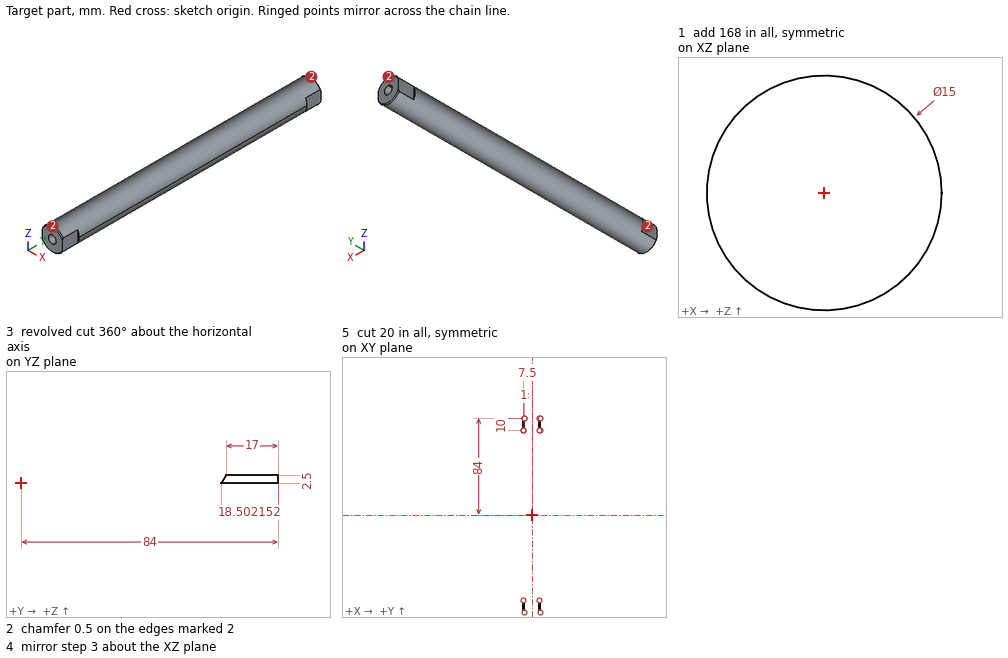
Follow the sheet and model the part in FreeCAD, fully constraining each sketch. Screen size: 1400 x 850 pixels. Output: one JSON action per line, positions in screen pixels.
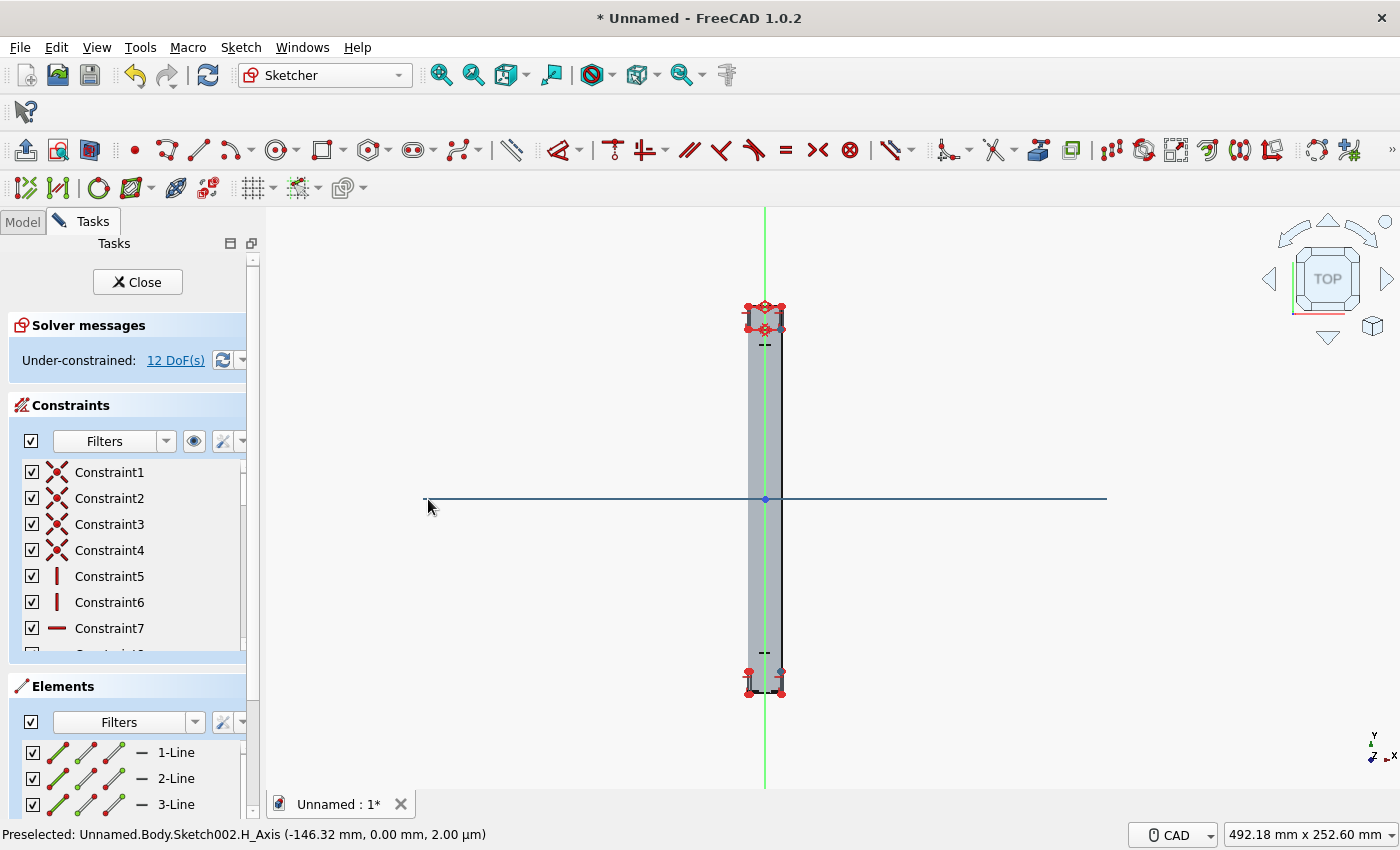
{"action": "left_click", "coordinate": [818, 150]}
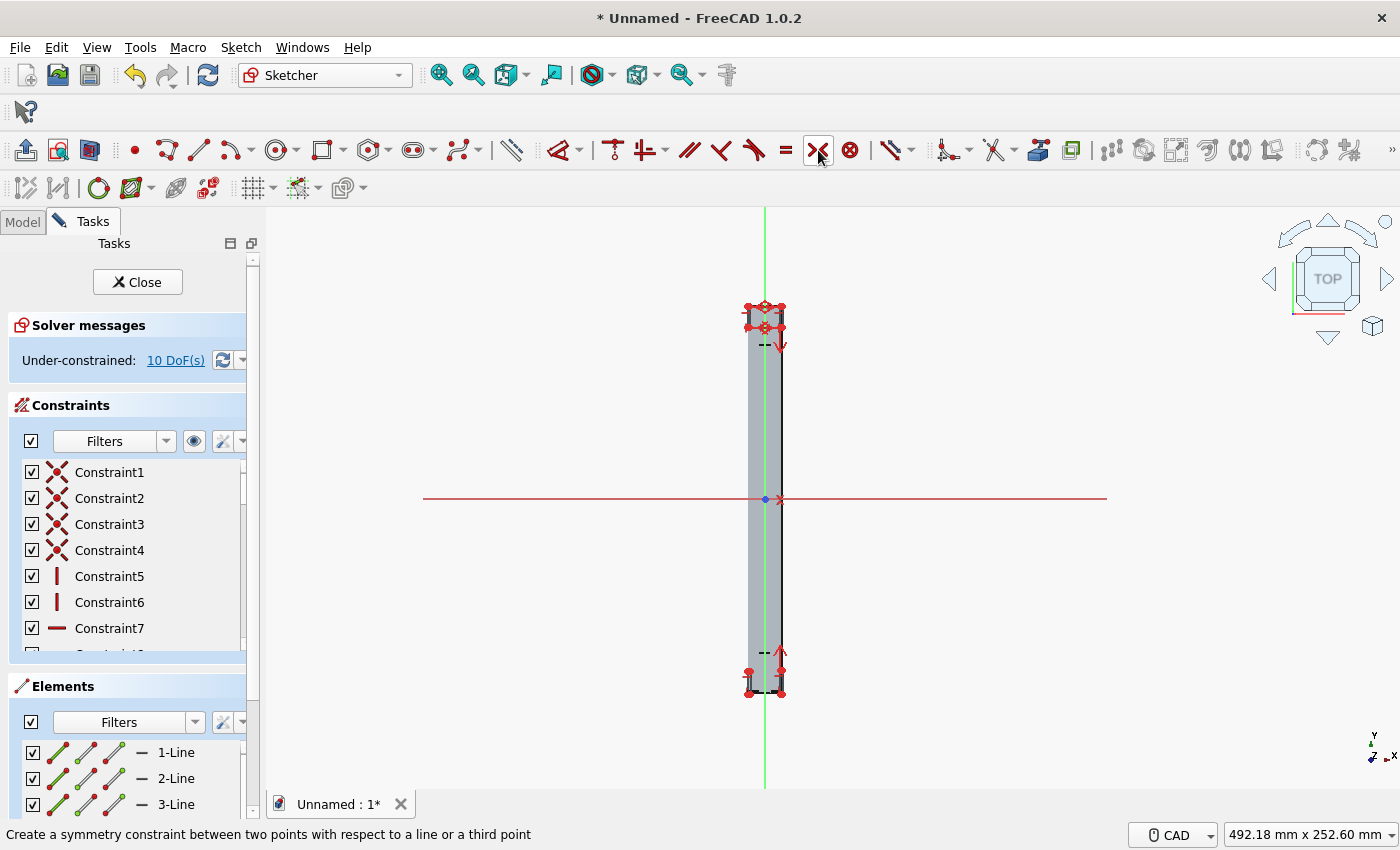
{"action": "scroll", "coordinate": [783, 307], "scroll_direction": "up", "scroll_amount": 9}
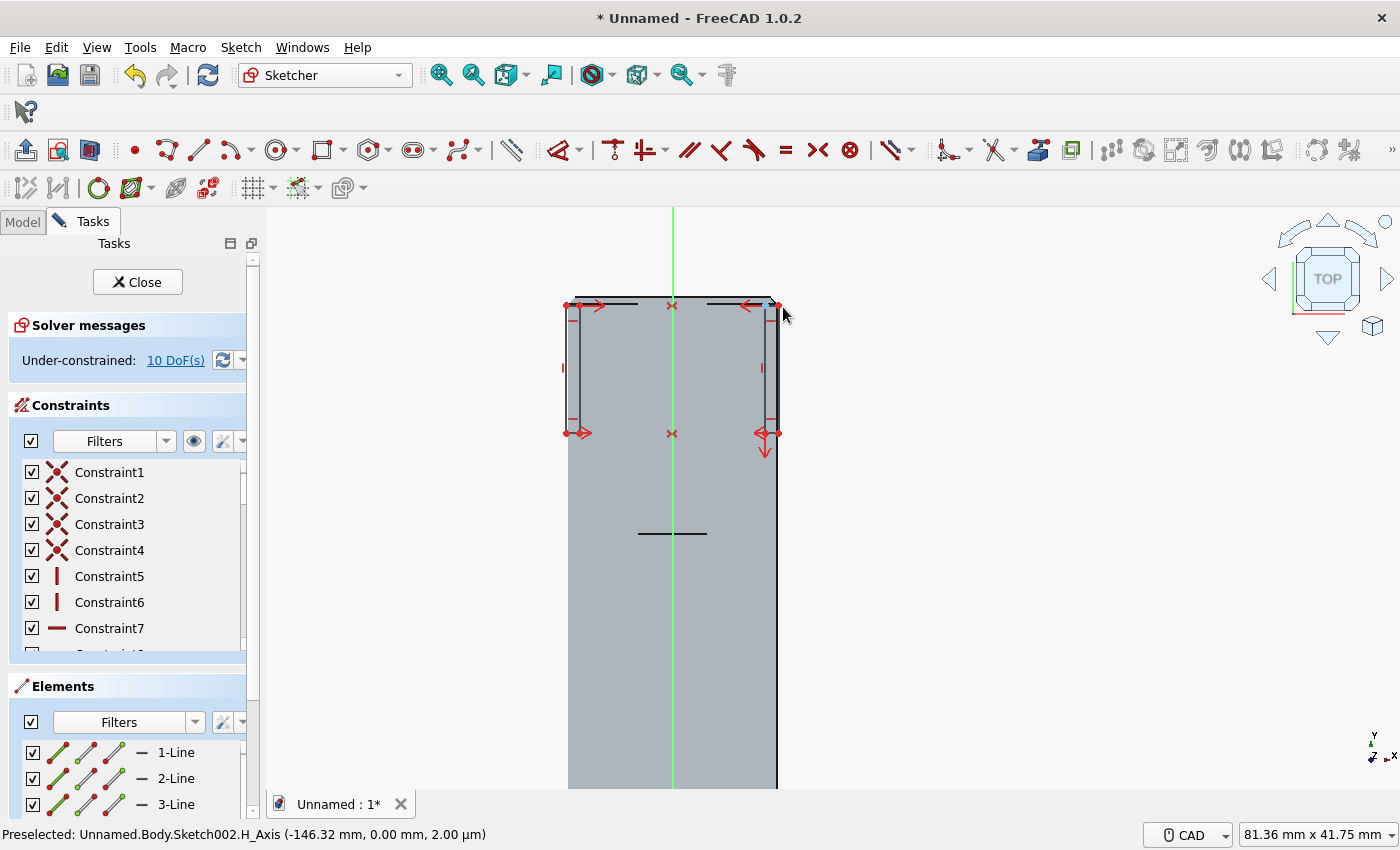
{"action": "left_click", "coordinate": [779, 306]}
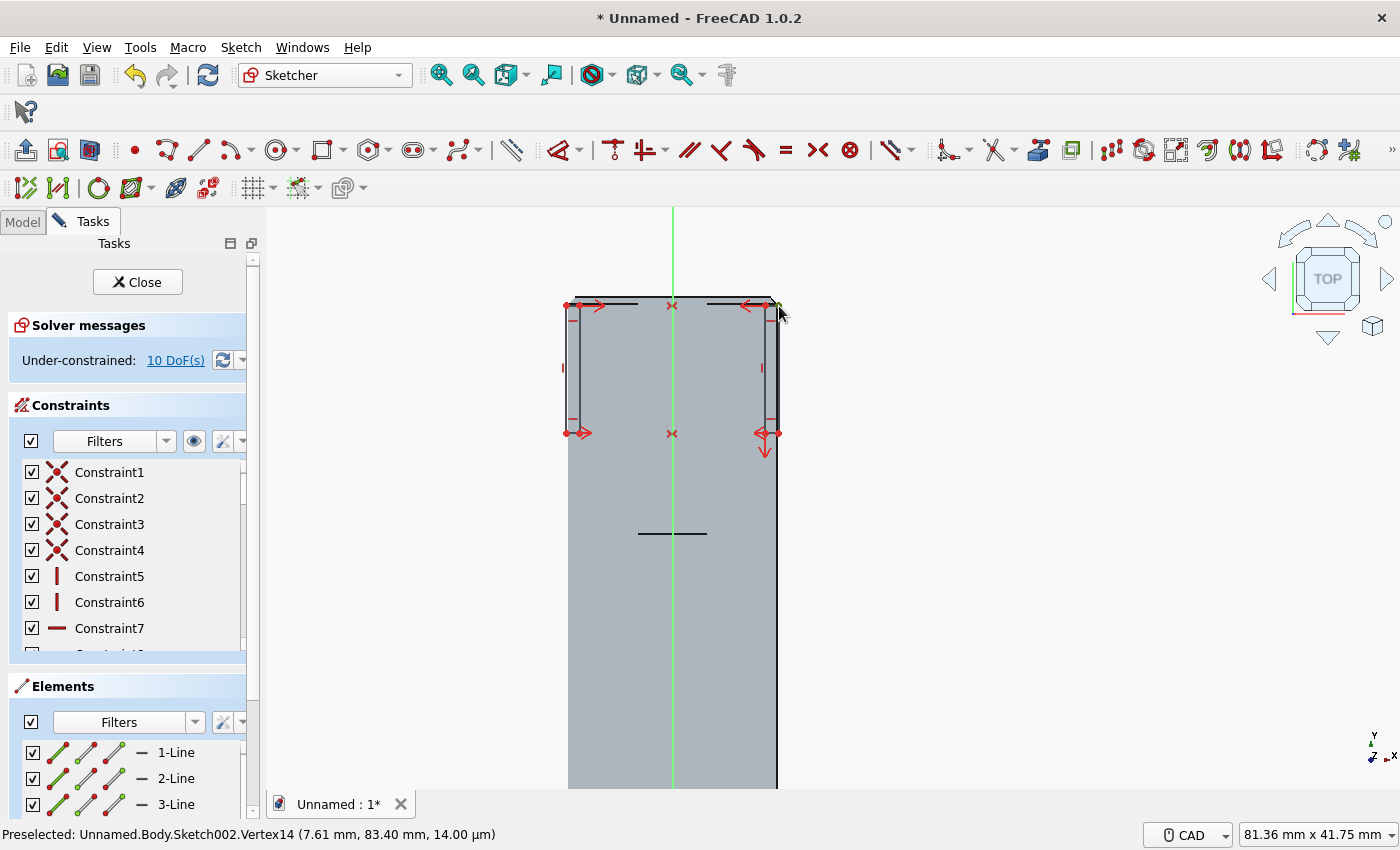
{"action": "scroll", "coordinate": [783, 306], "scroll_direction": "down", "scroll_amount": 9}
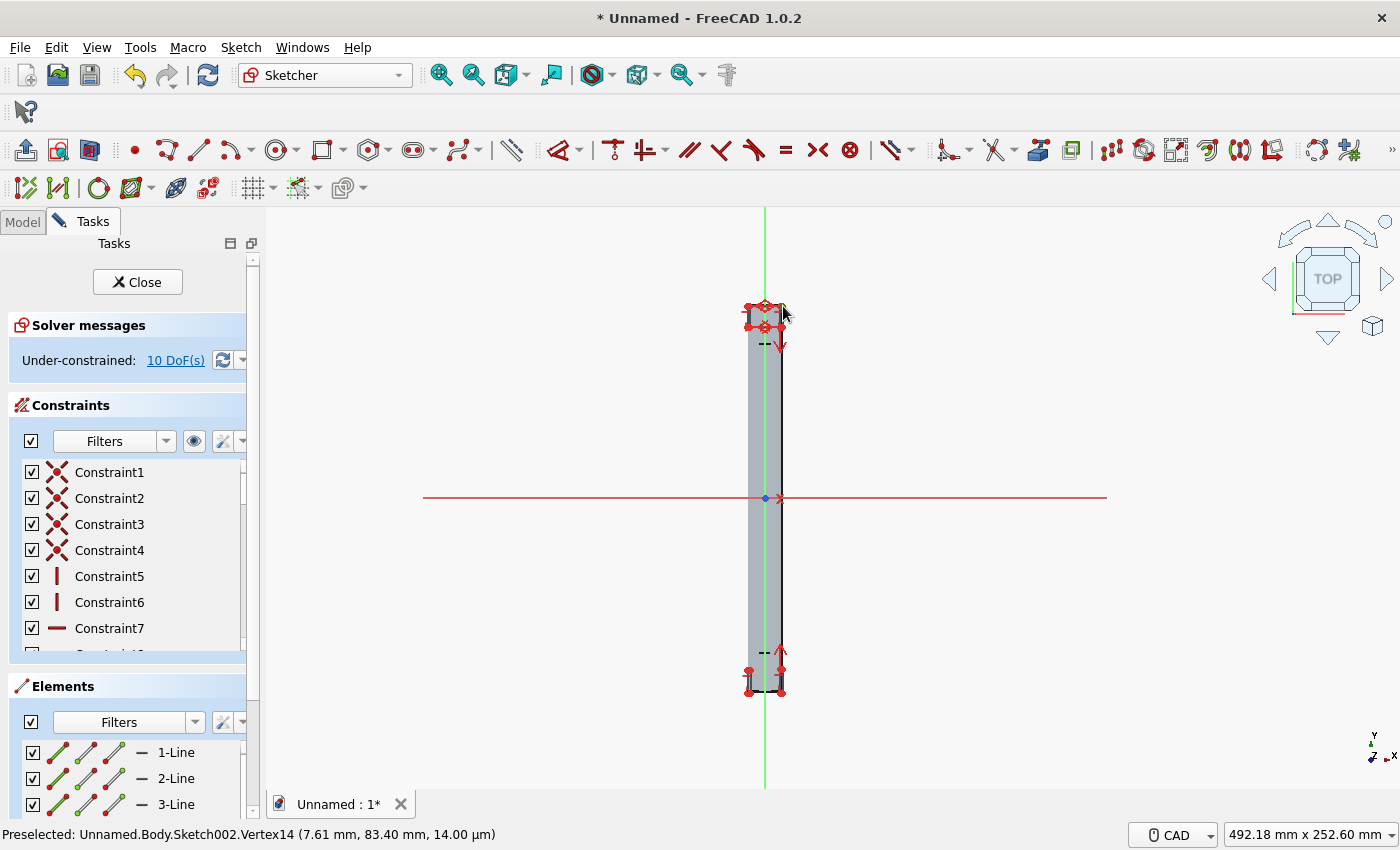
{"action": "scroll", "coordinate": [783, 693], "scroll_direction": "up", "scroll_amount": 9}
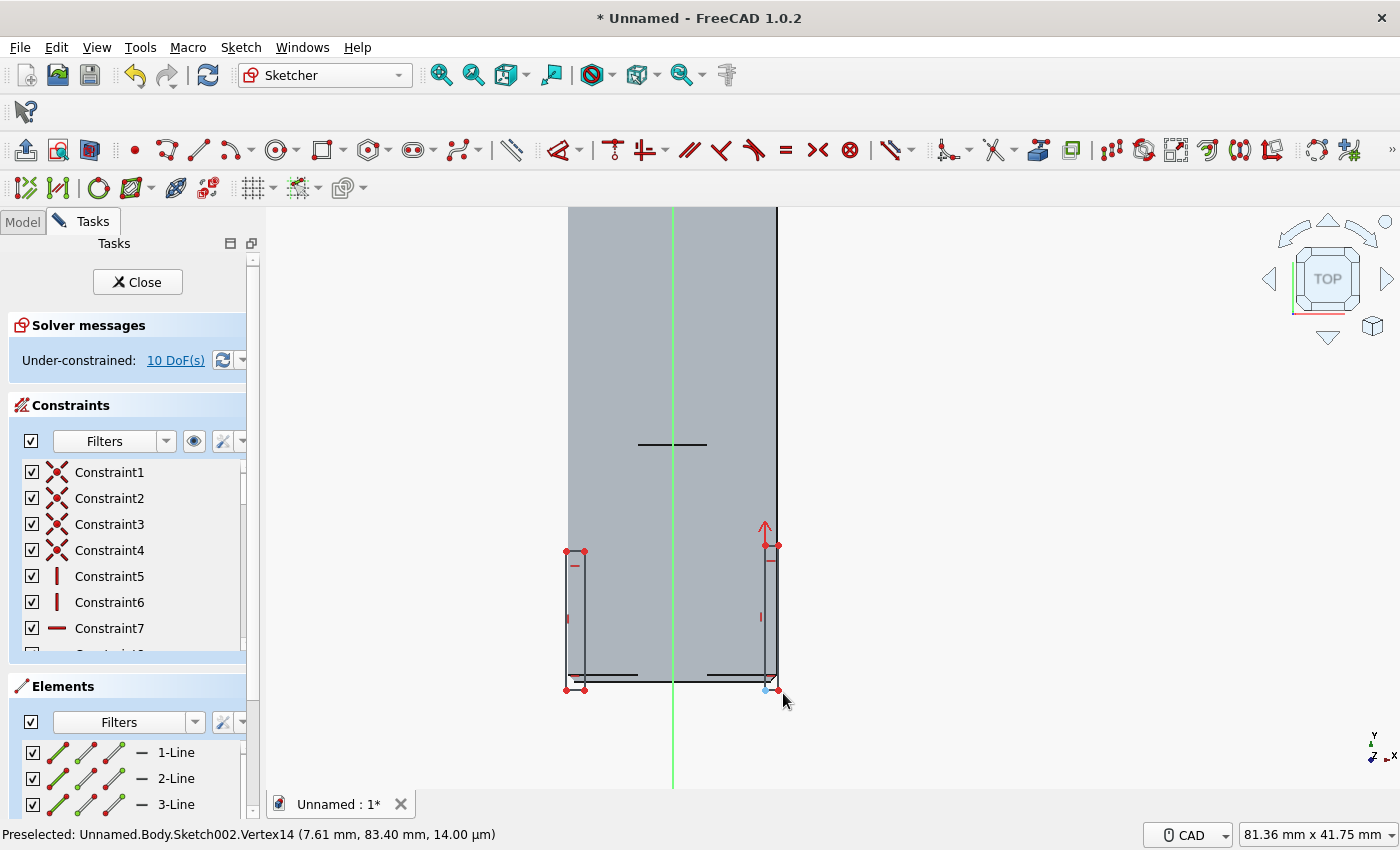
{"action": "left_click", "coordinate": [778, 690]}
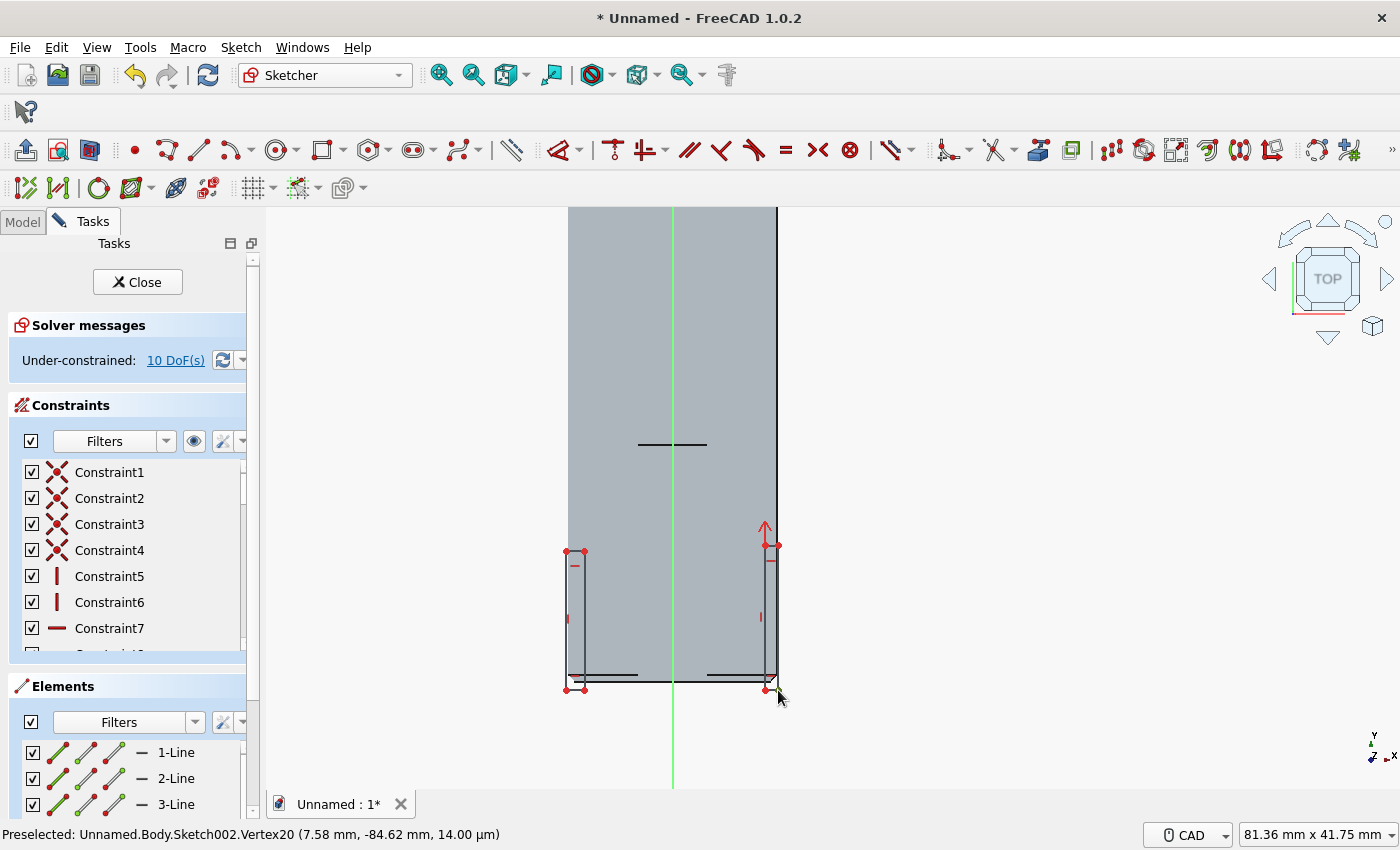
{"action": "scroll", "coordinate": [783, 694], "scroll_direction": "down", "scroll_amount": 9}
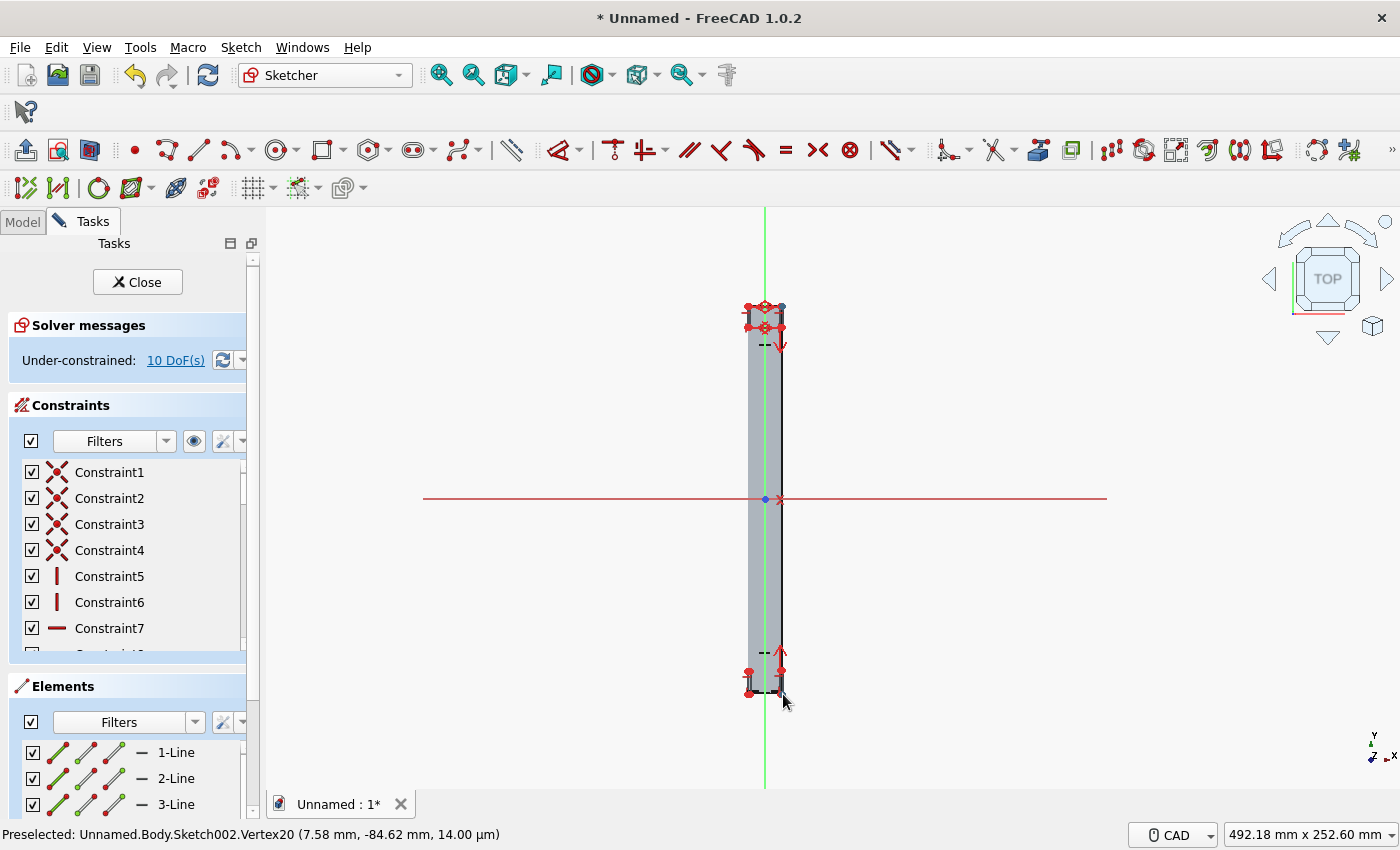
{"action": "left_click", "coordinate": [428, 499]}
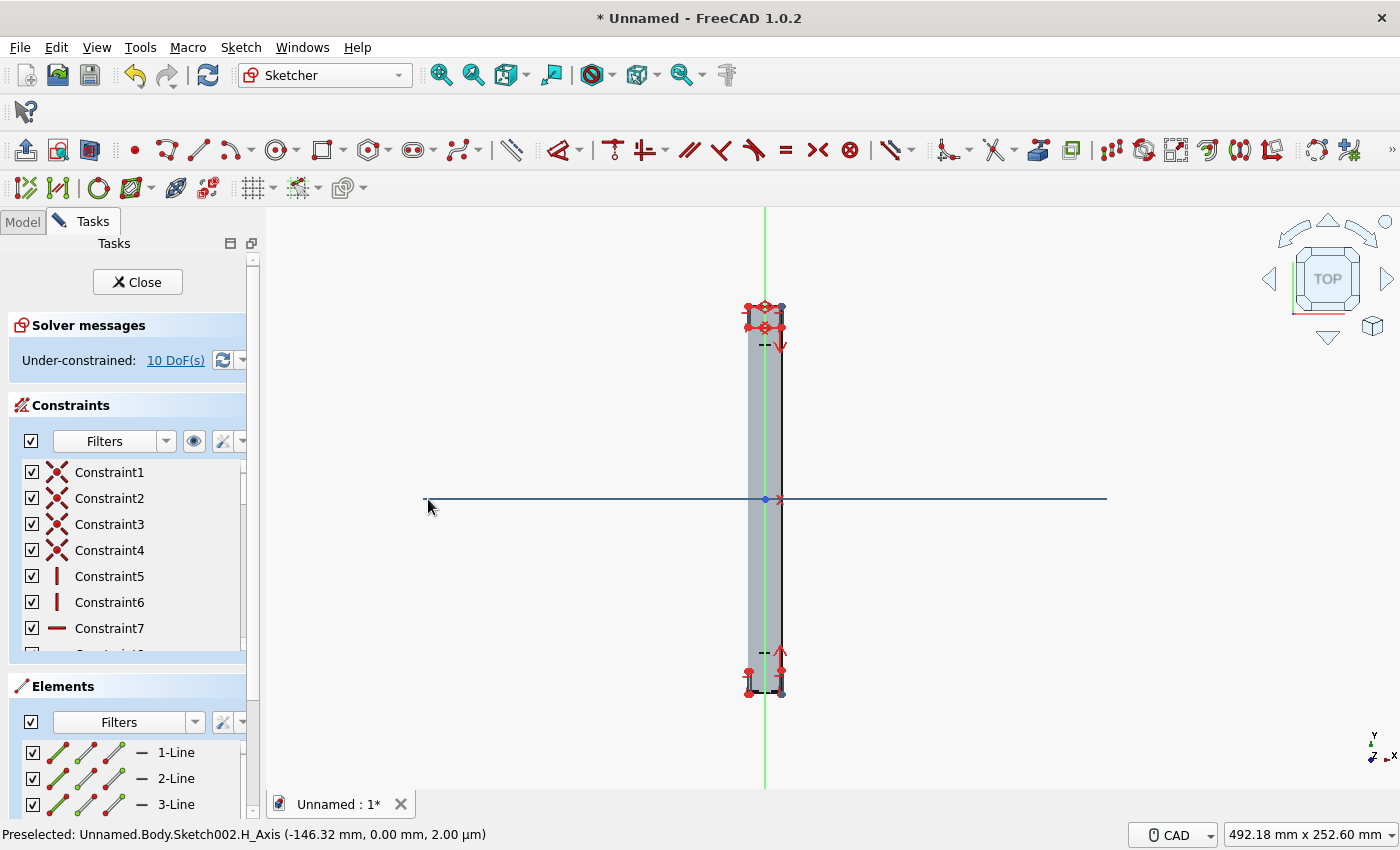
{"action": "left_click", "coordinate": [818, 150]}